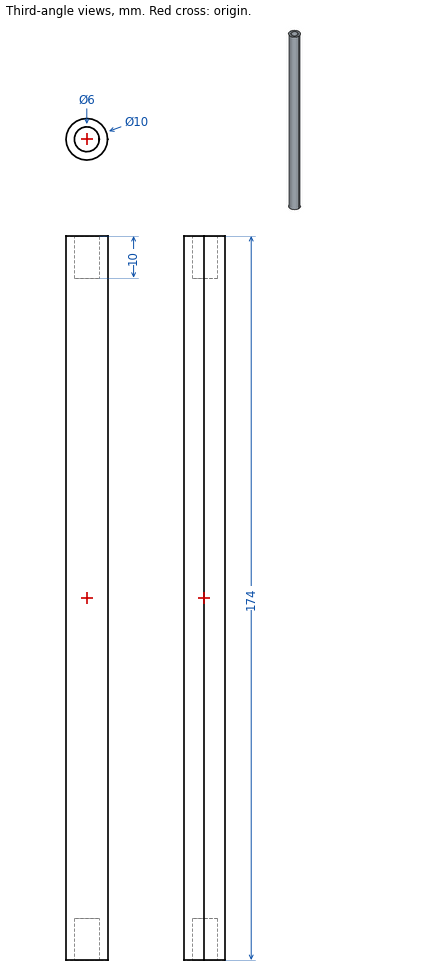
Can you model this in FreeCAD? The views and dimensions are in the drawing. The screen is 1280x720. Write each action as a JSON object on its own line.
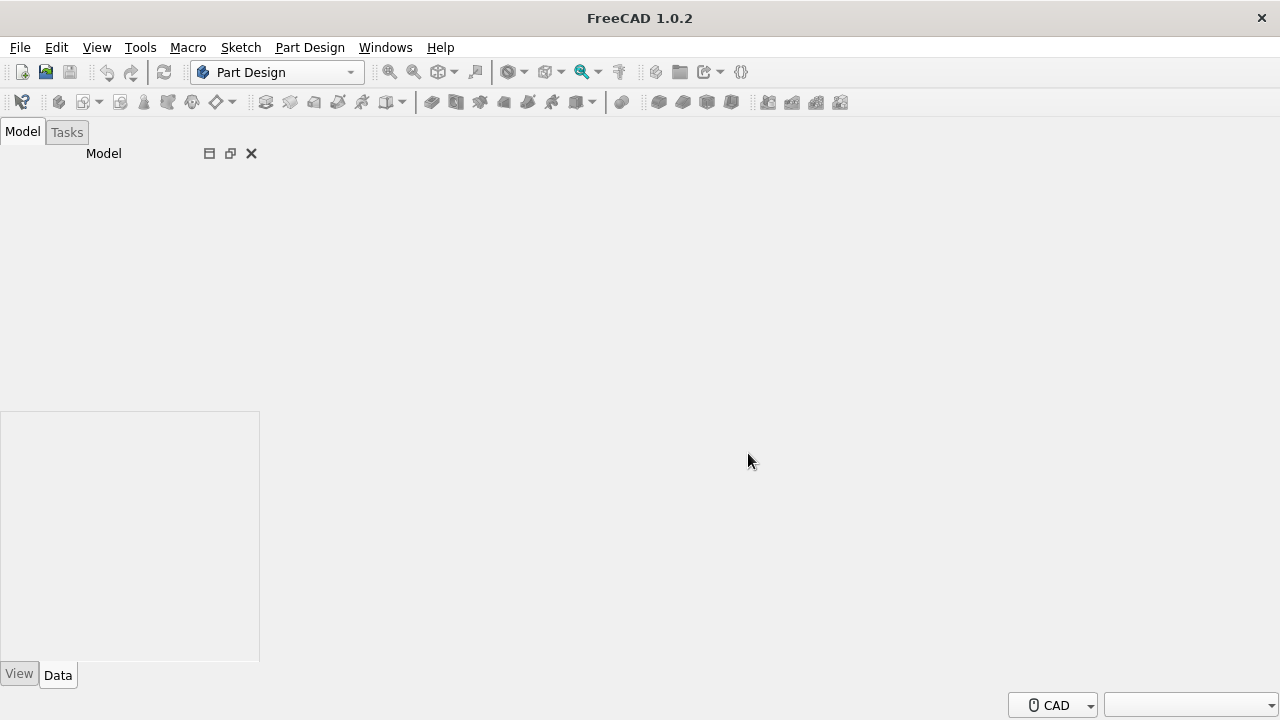
{"action": "left_click", "coordinate": [22, 72]}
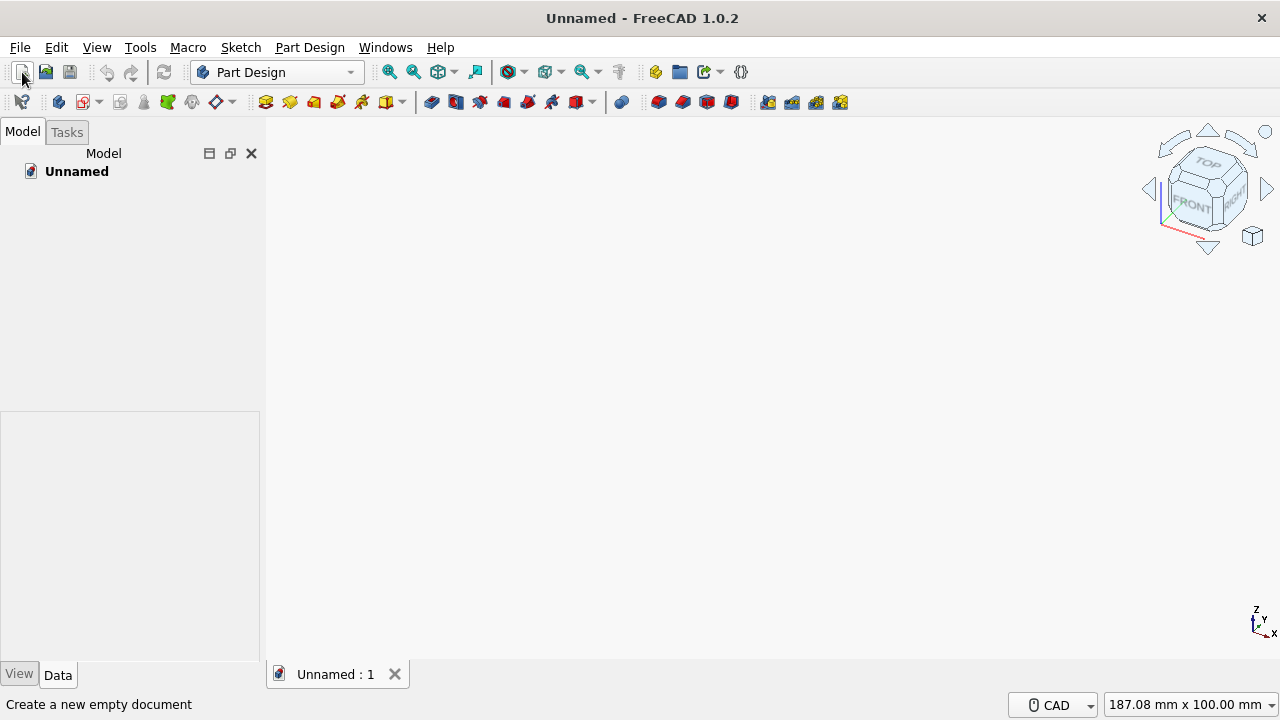
{"action": "left_click", "coordinate": [84, 102]}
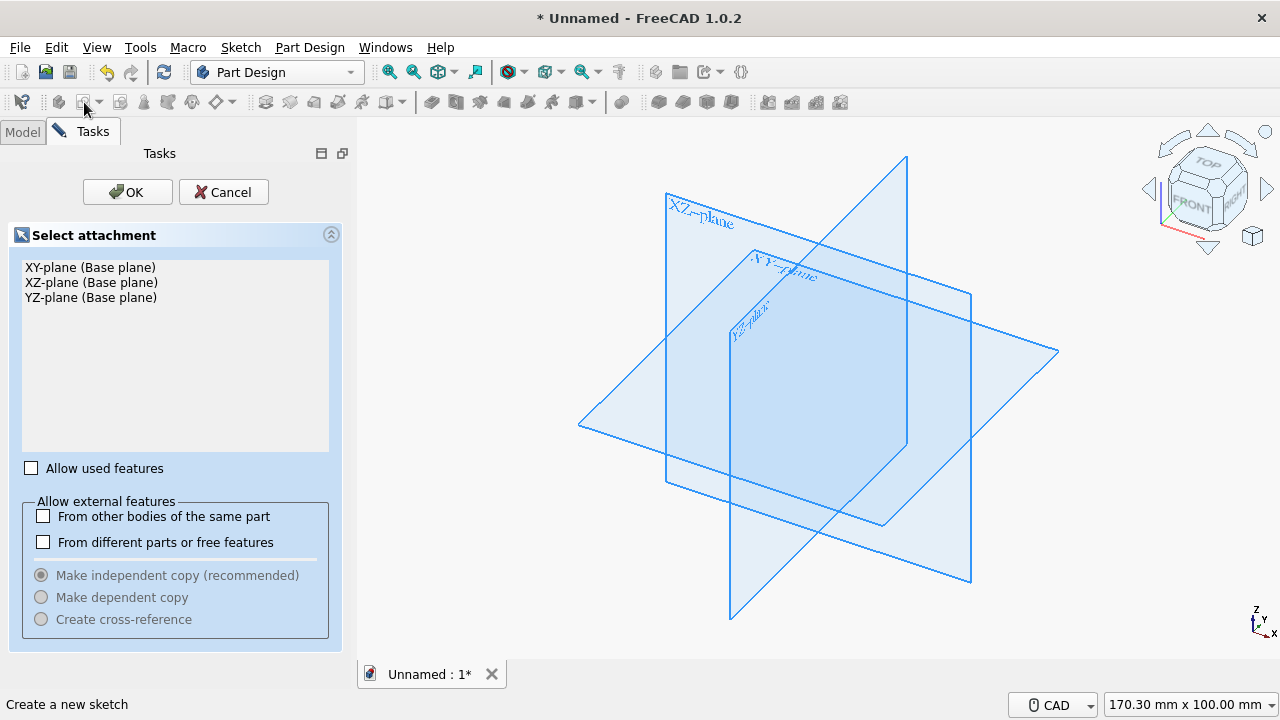
{"action": "left_click", "coordinate": [82, 268]}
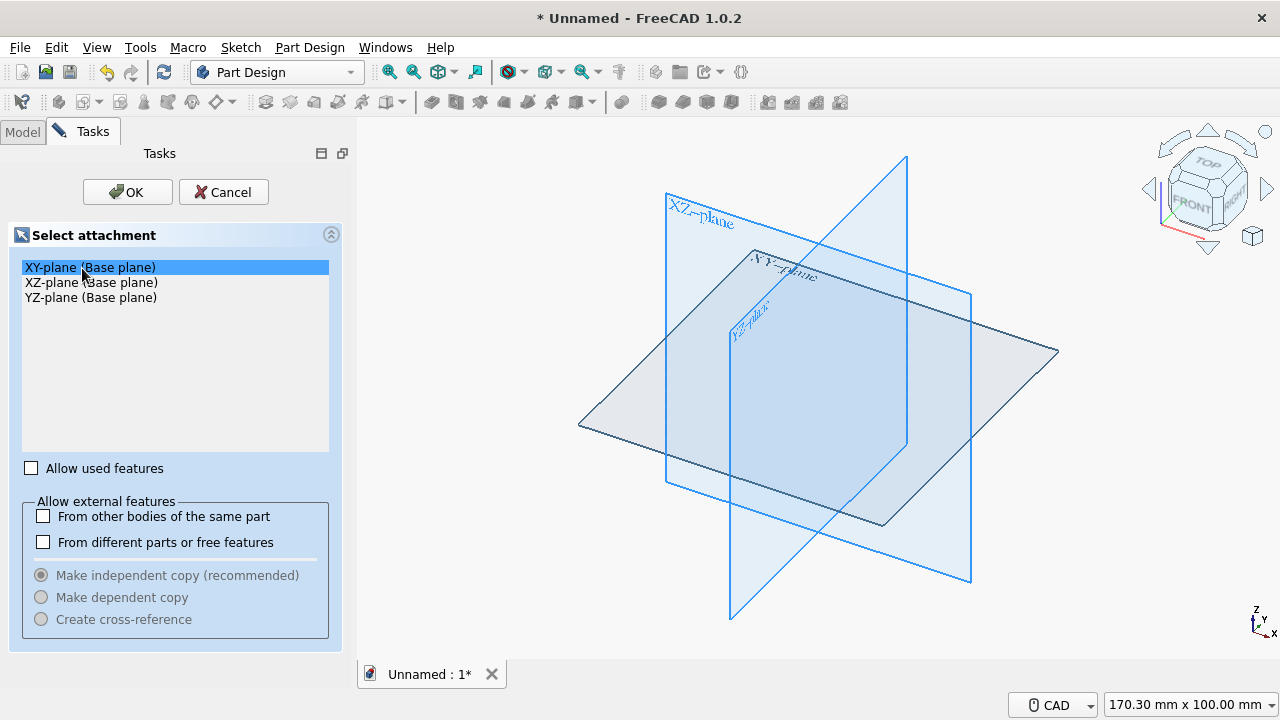
{"action": "left_click", "coordinate": [128, 192]}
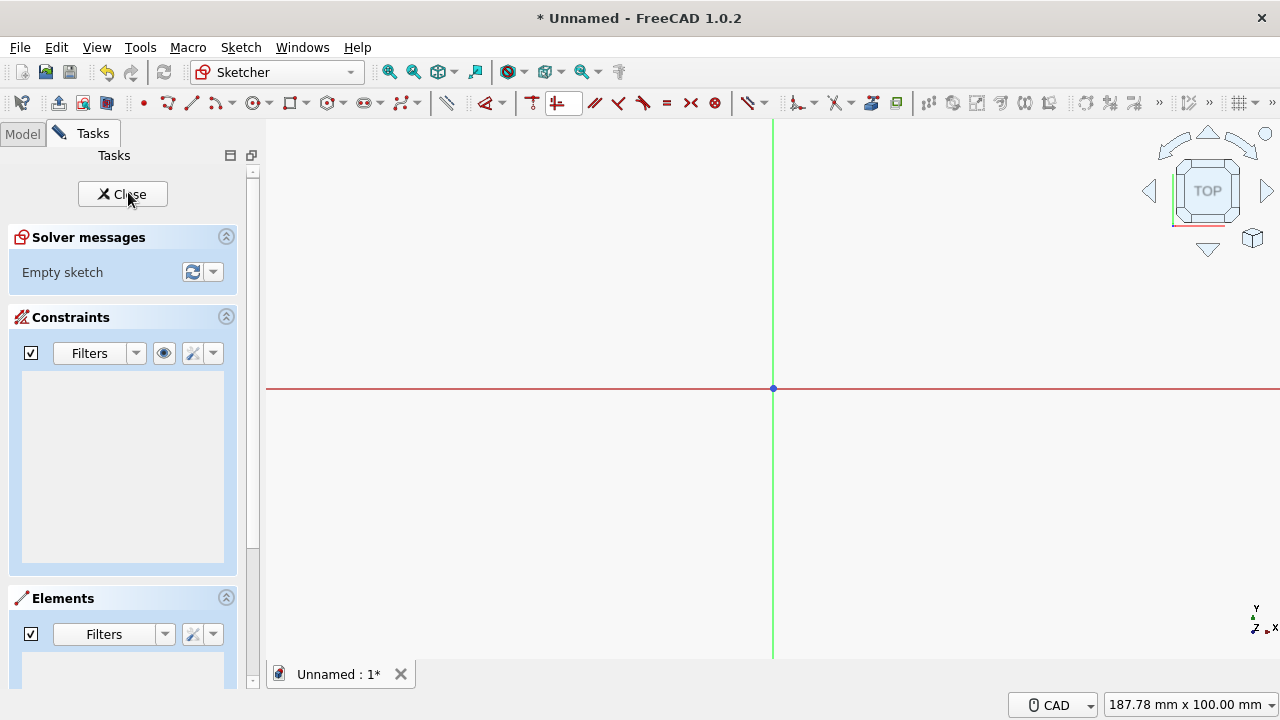
{"action": "scroll", "coordinate": [787, 389], "scroll_direction": "up", "scroll_amount": 9}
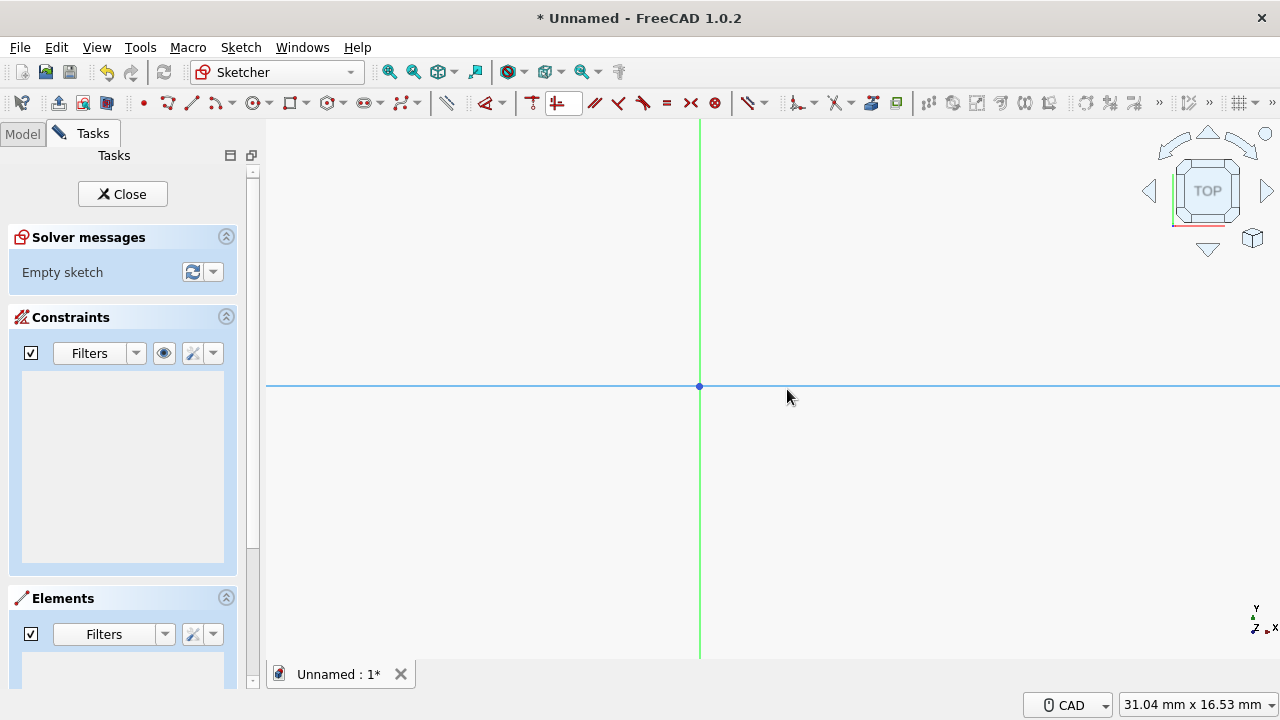
{"action": "left_click", "coordinate": [254, 104]}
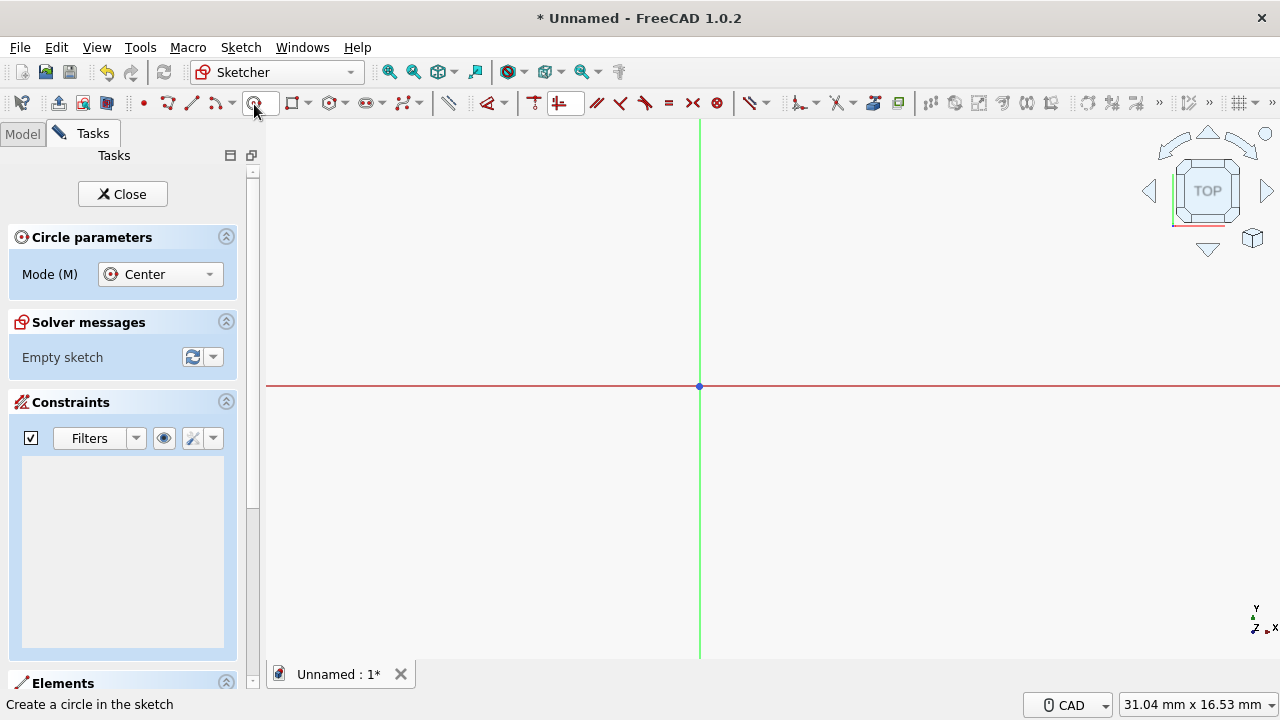
{"action": "left_click", "coordinate": [700, 386]}
{"action": "left_click", "coordinate": [815, 271]}
{"action": "key", "text": "Escape"}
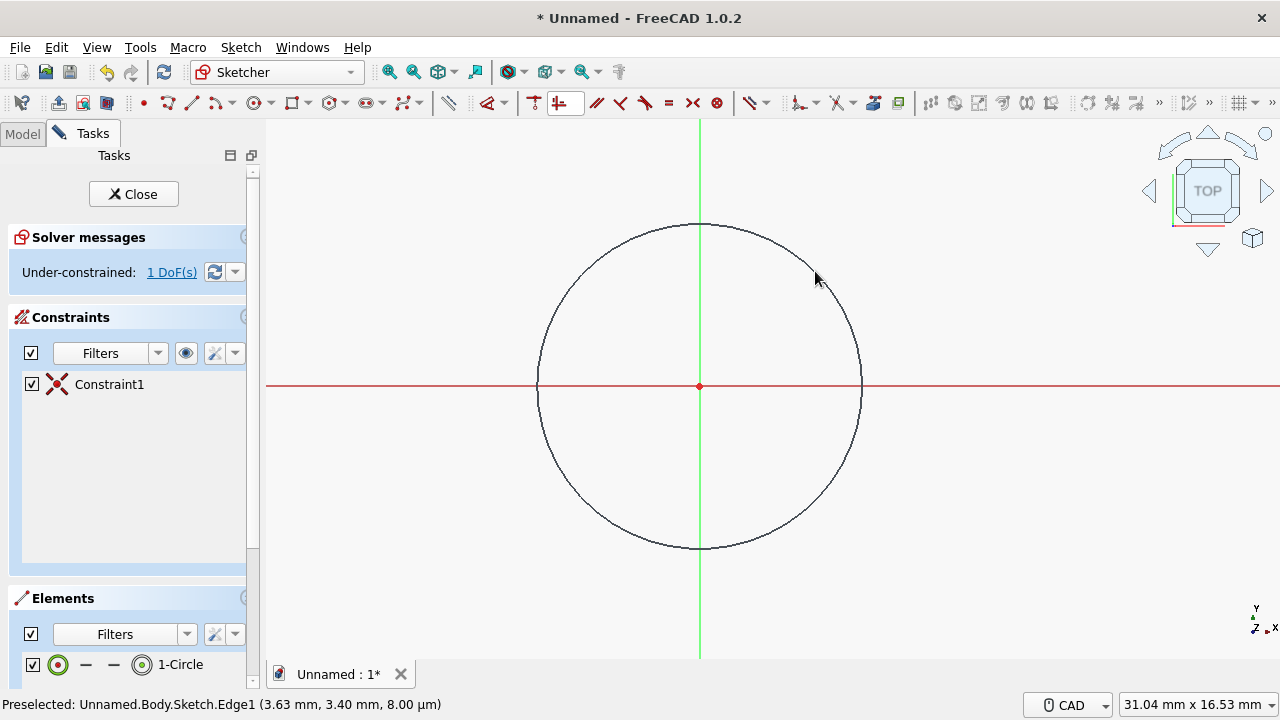
{"action": "left_click", "coordinate": [488, 104]}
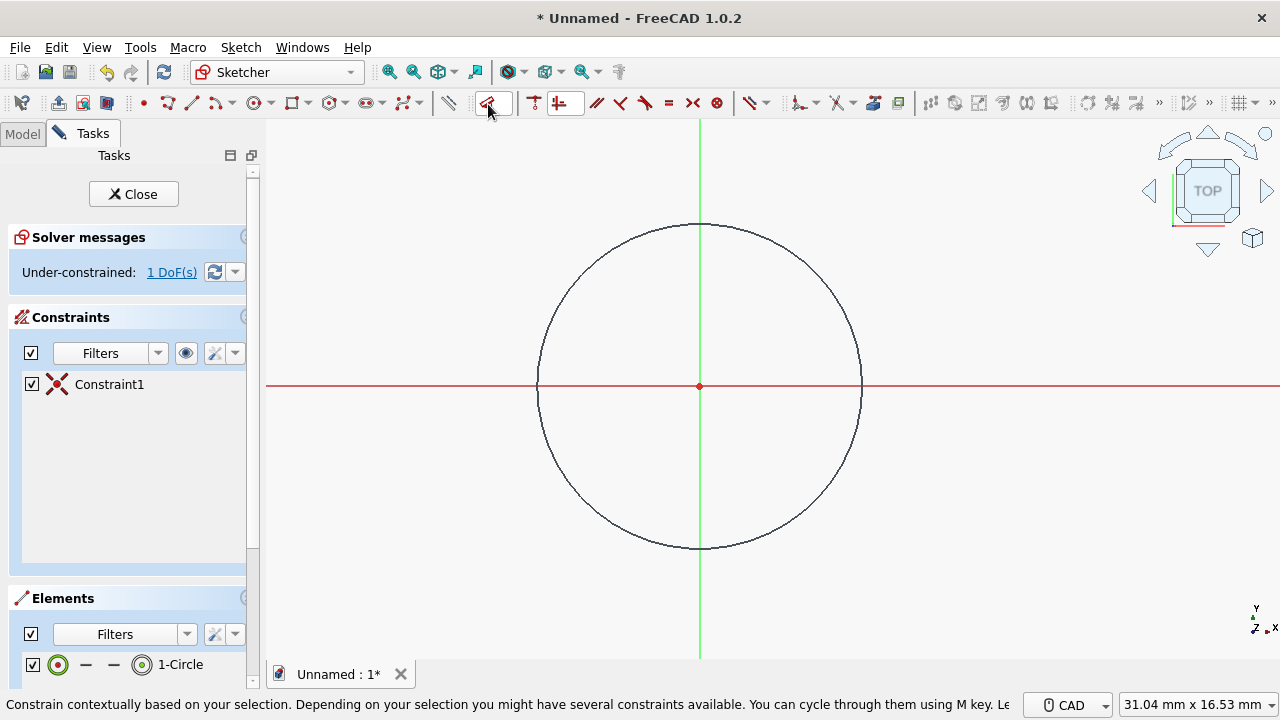
{"action": "left_click", "coordinate": [814, 271]}
{"action": "left_click", "coordinate": [837, 248]}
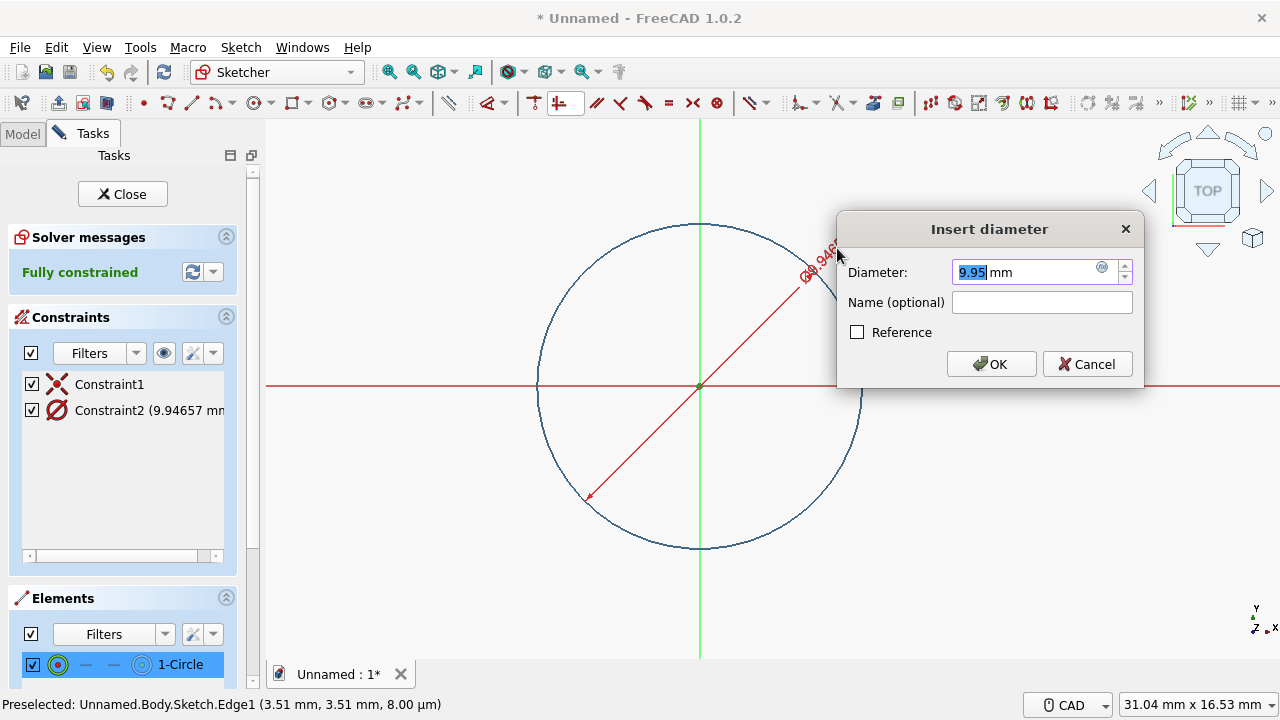
{"action": "type", "text": "10"}
{"action": "key", "text": "Return"}
{"action": "key", "text": "Escape"}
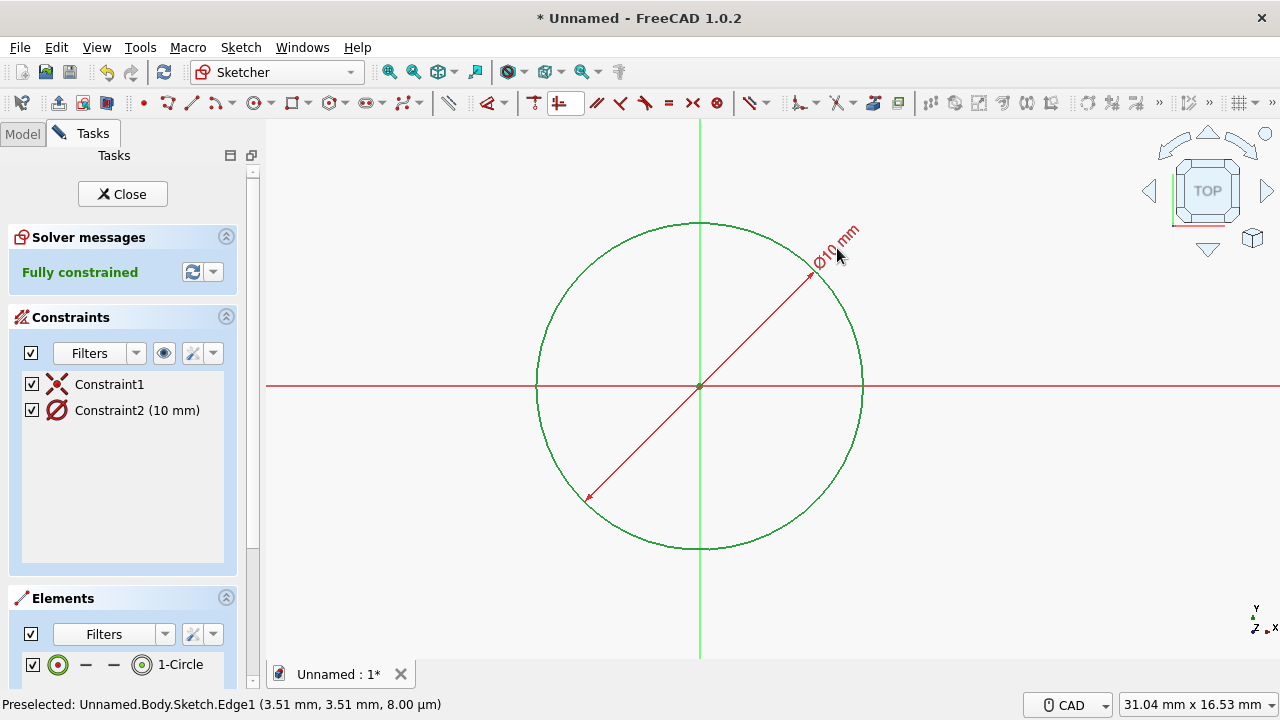
{"action": "left_click", "coordinate": [123, 194]}